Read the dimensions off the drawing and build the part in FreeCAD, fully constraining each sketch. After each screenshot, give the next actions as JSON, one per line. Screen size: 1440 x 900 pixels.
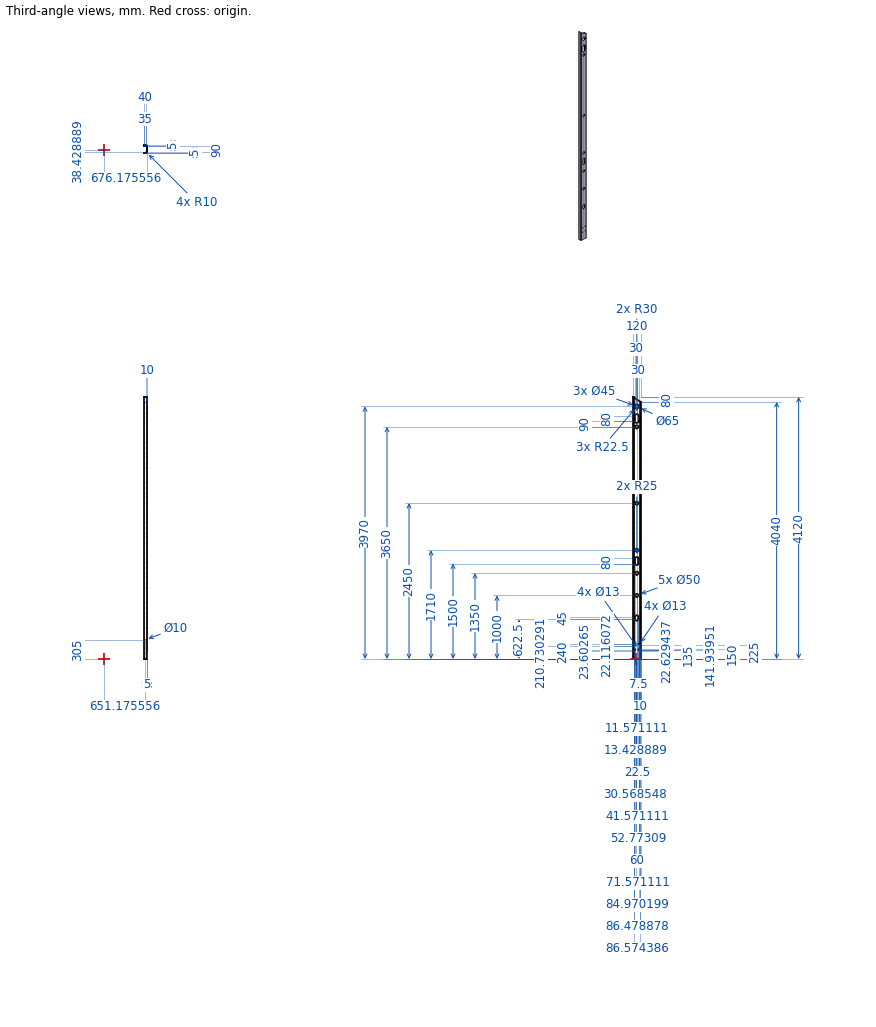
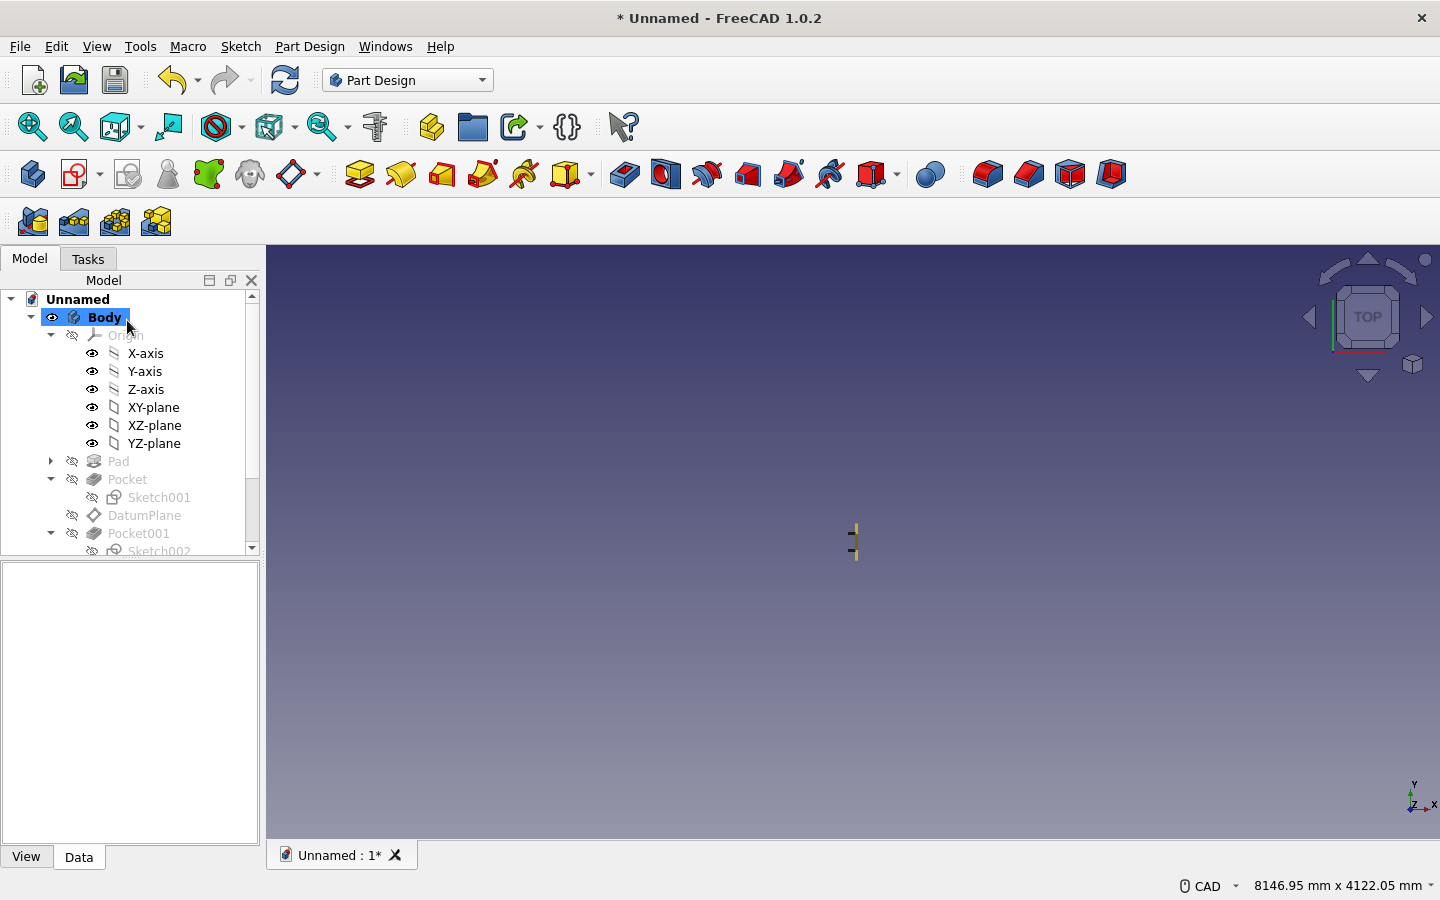
{"action": "scroll", "coordinate": [101, 421], "scroll_direction": "down", "scroll_amount": 3}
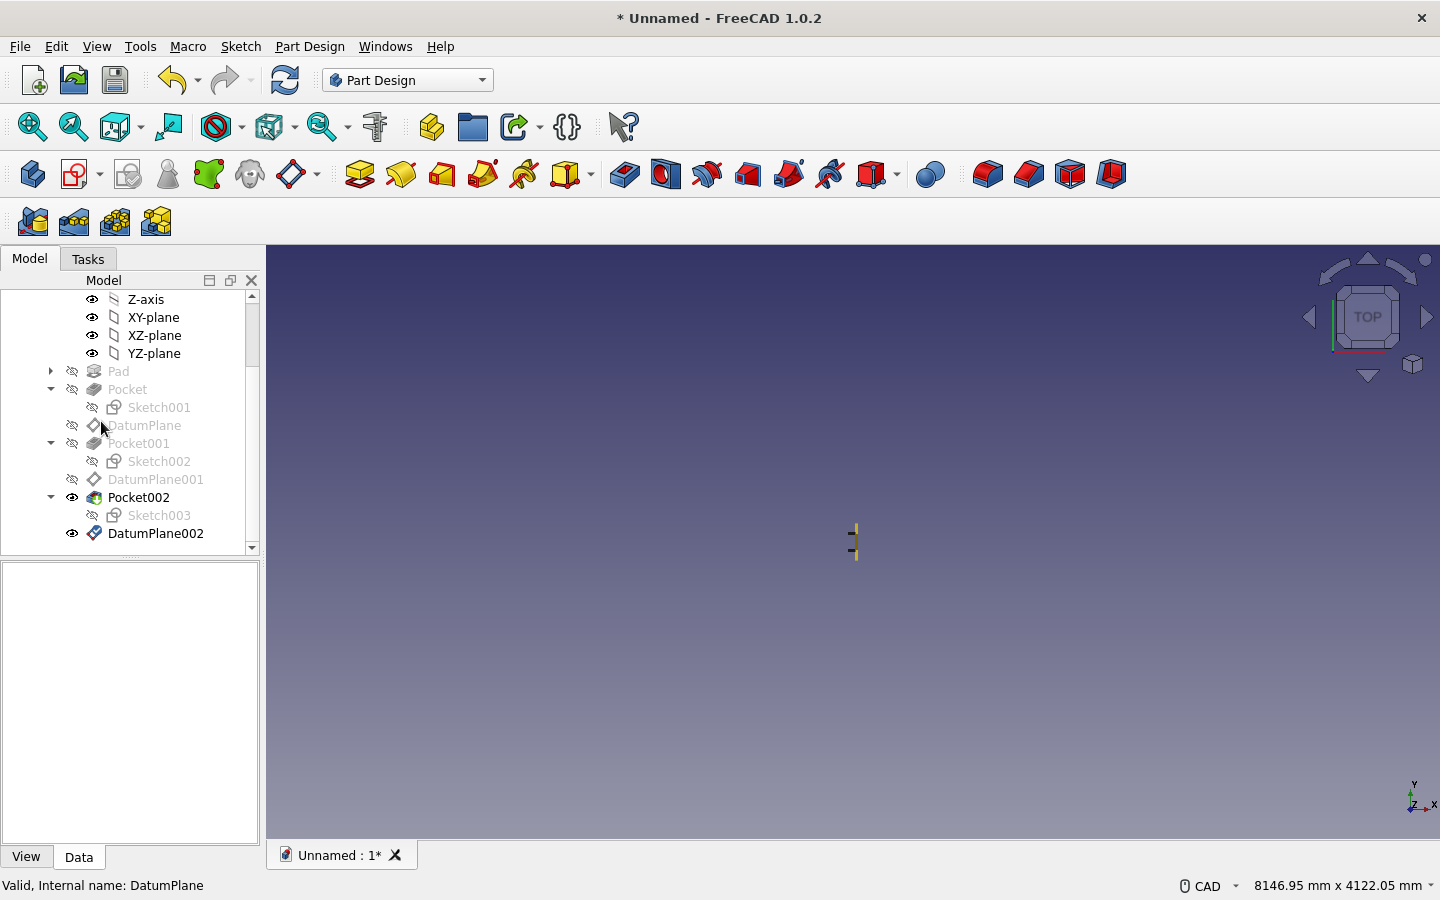
{"action": "left_click", "coordinate": [117, 533]}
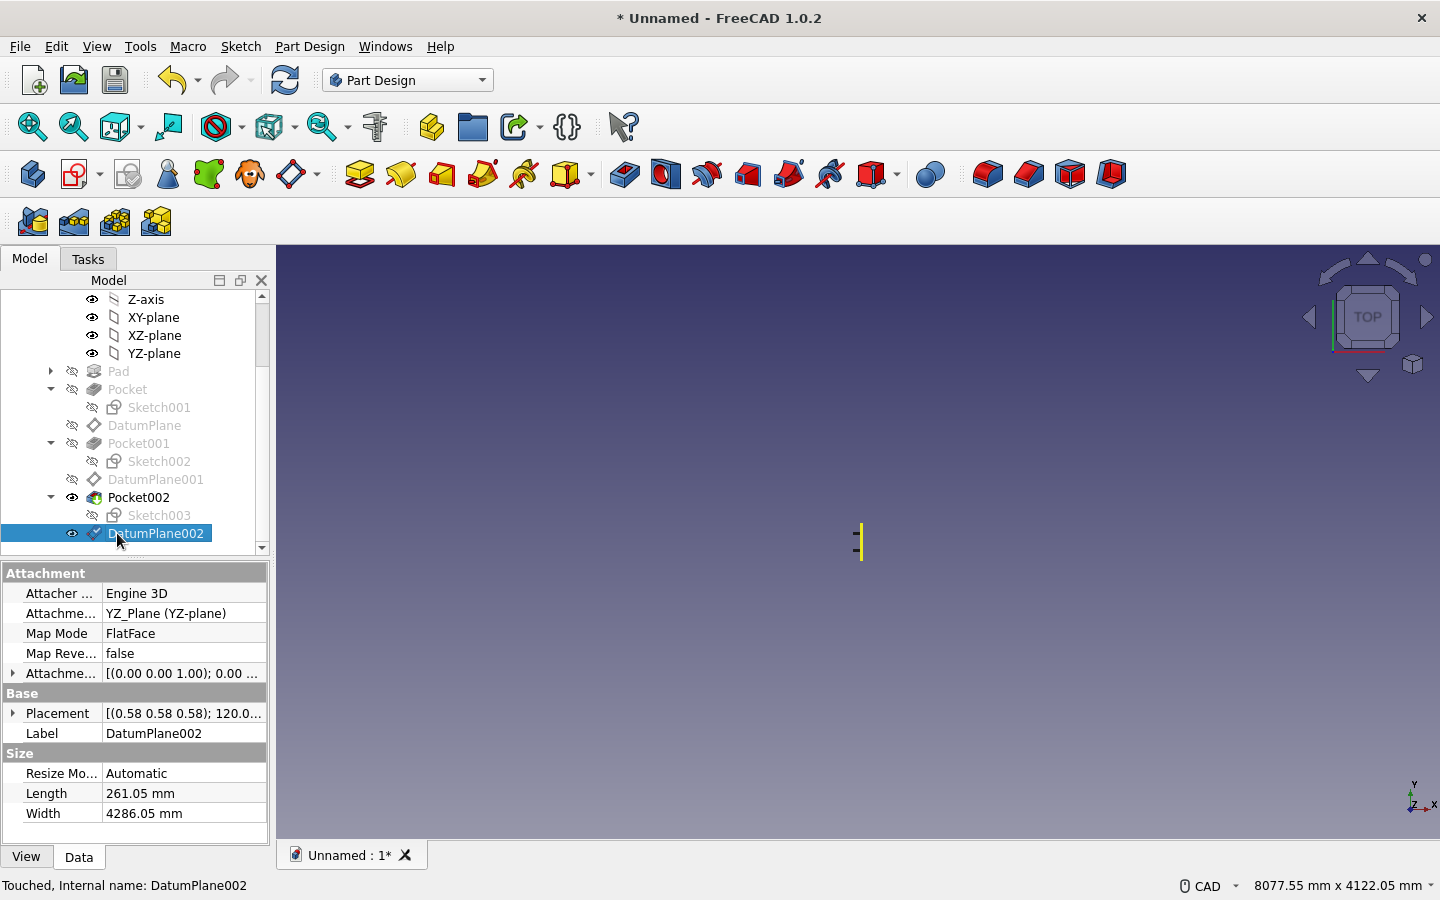
{"action": "left_click", "coordinate": [74, 174]}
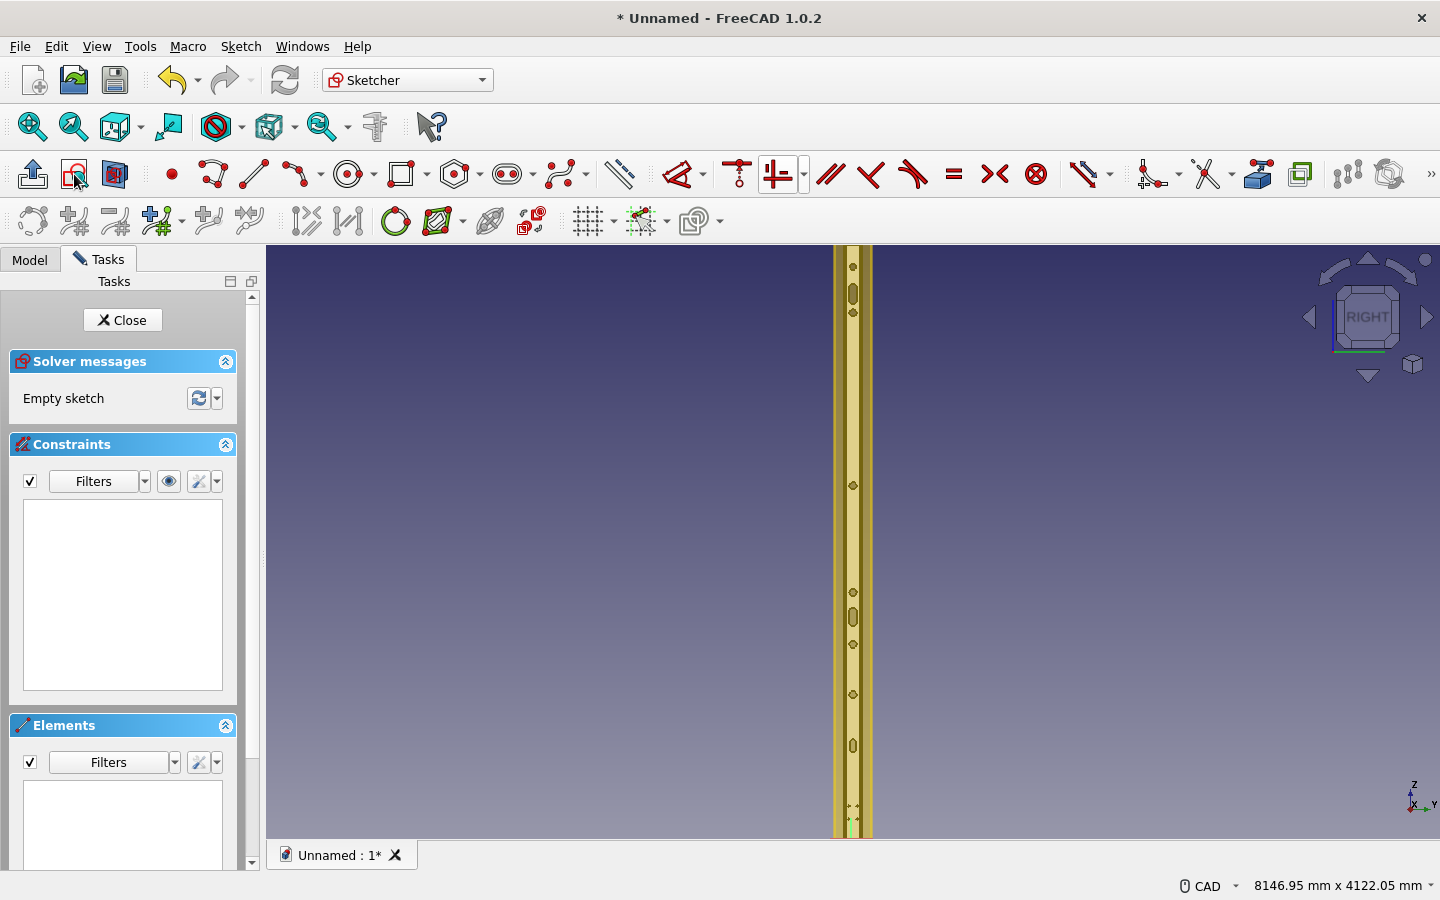
{"action": "scroll", "coordinate": [784, 542], "scroll_direction": "down", "scroll_amount": 5}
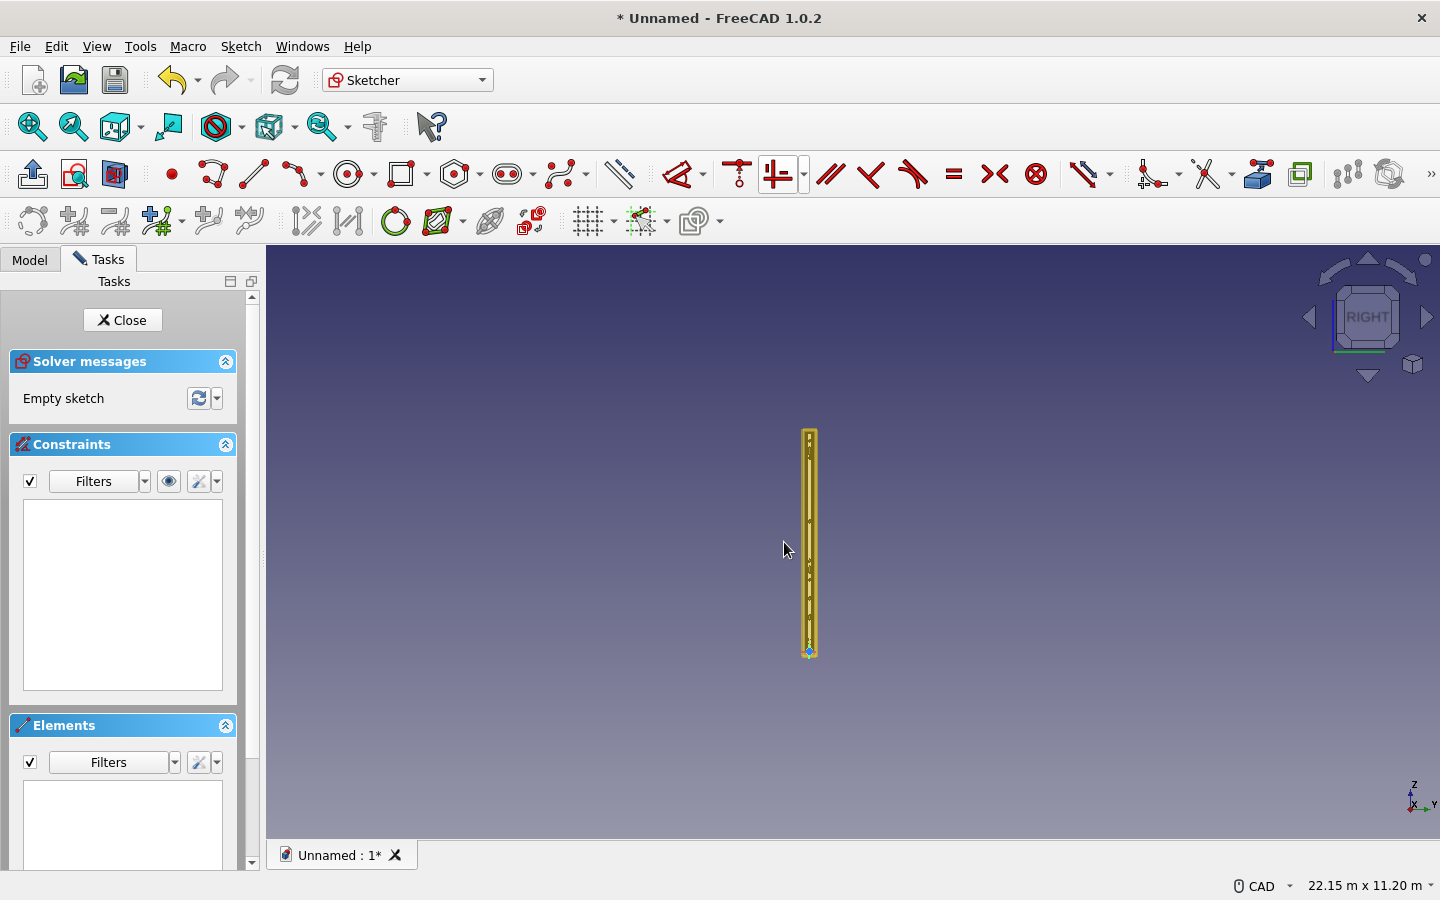
{"action": "scroll", "coordinate": [811, 650], "scroll_direction": "up", "scroll_amount": 15}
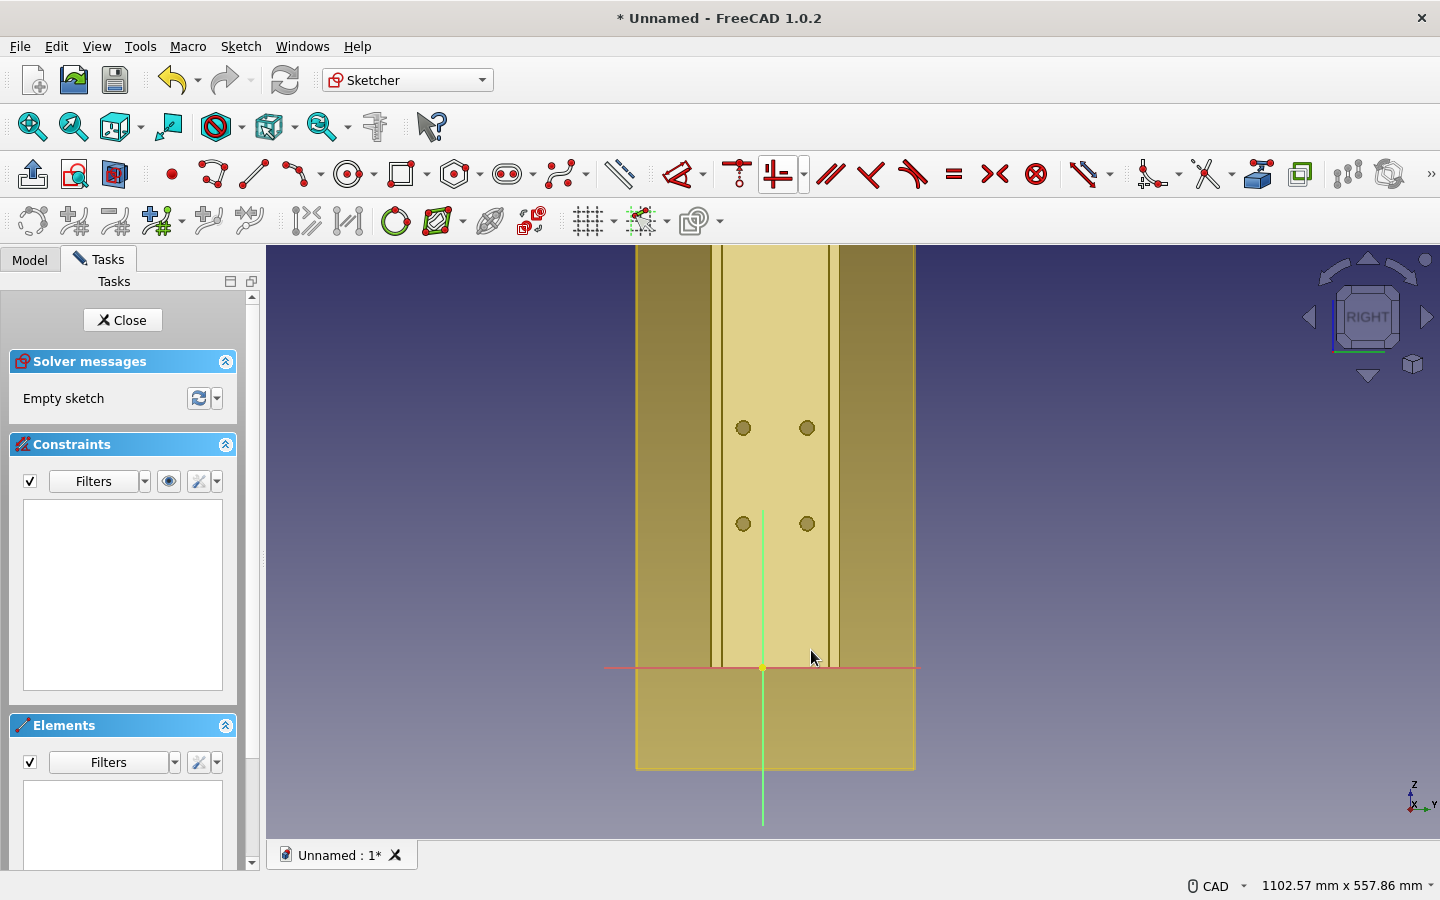
{"action": "scroll", "coordinate": [757, 525], "scroll_direction": "up", "scroll_amount": 2}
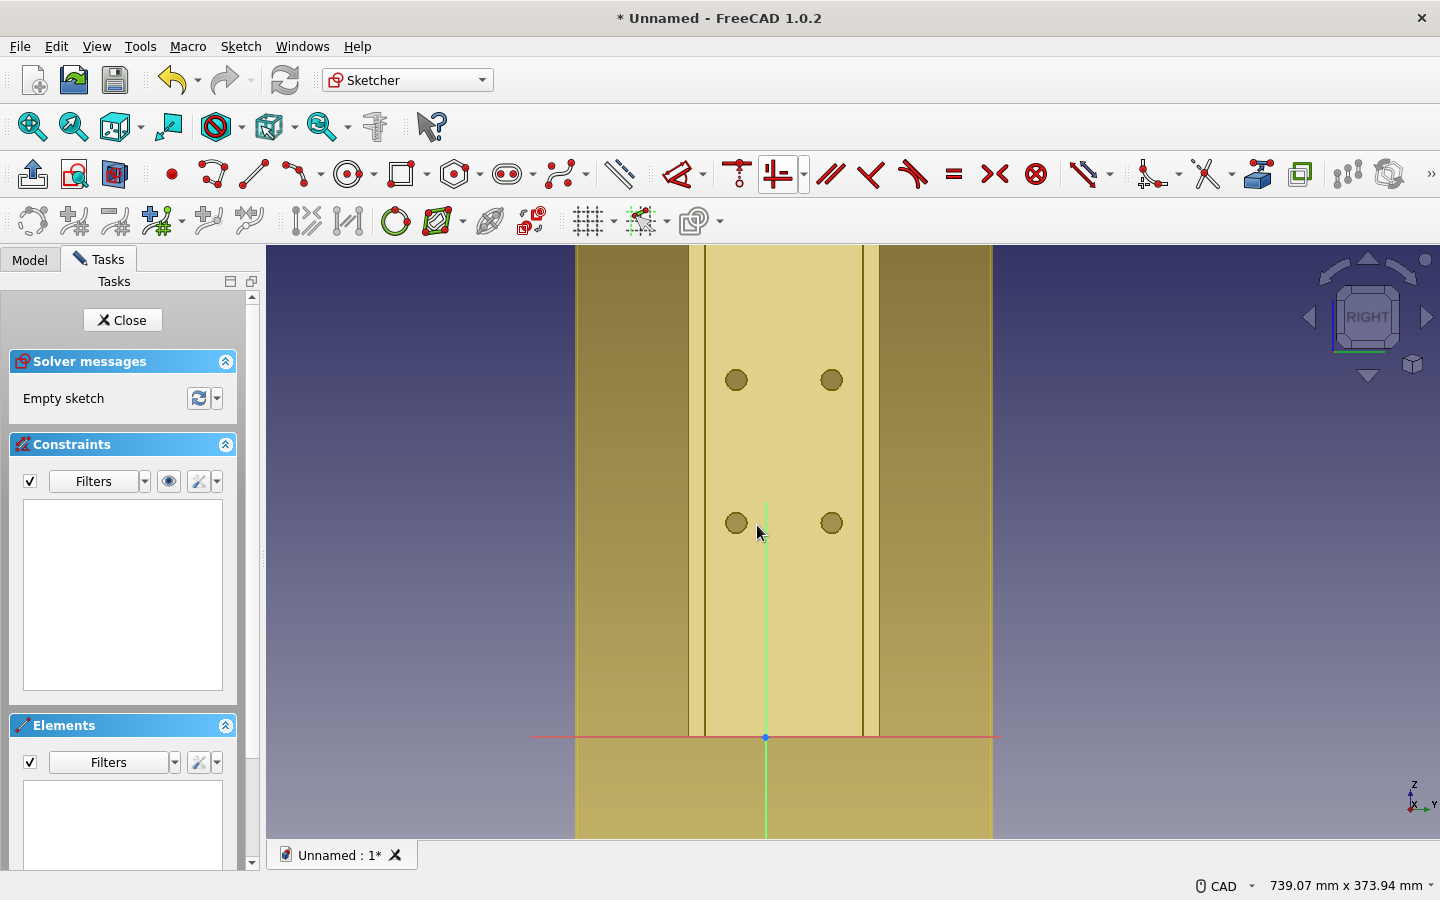
{"action": "key", "text": "g c"}